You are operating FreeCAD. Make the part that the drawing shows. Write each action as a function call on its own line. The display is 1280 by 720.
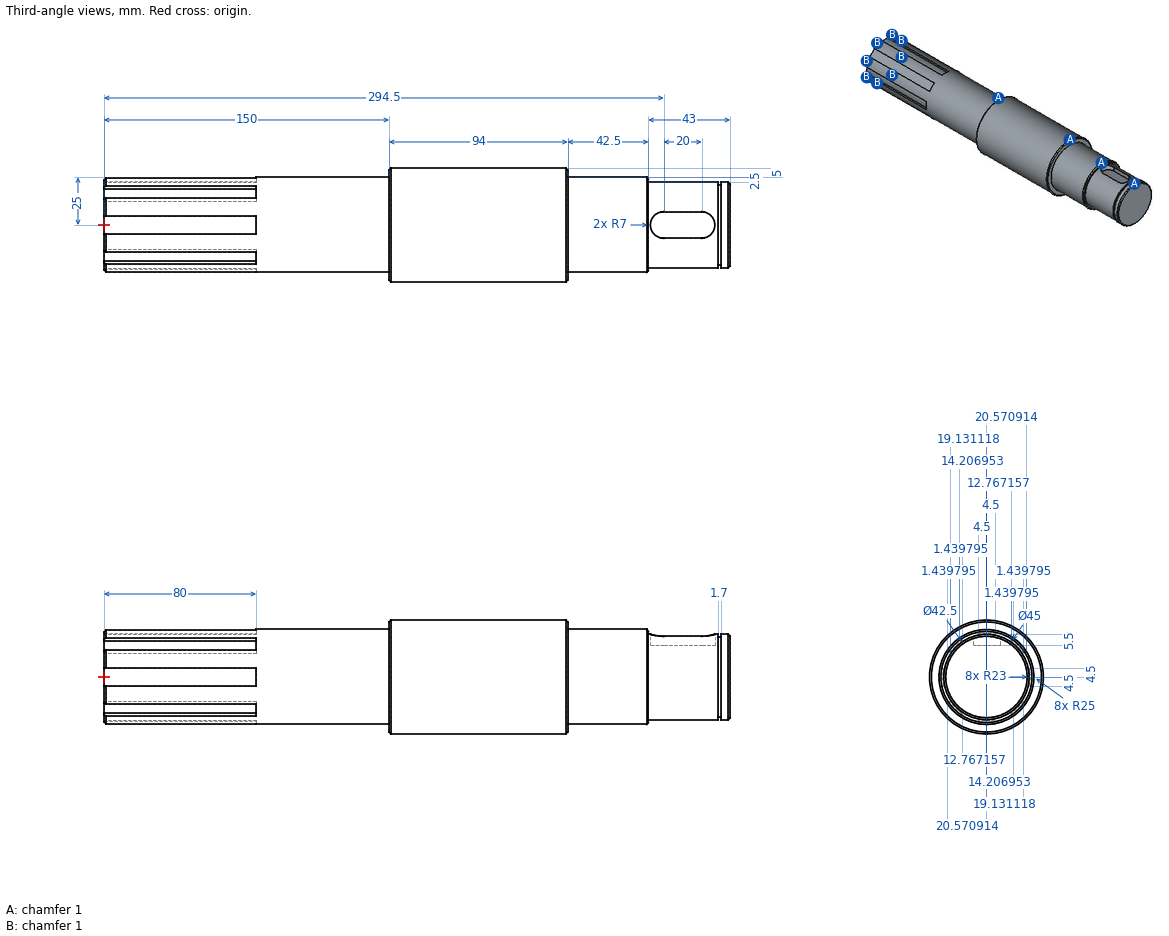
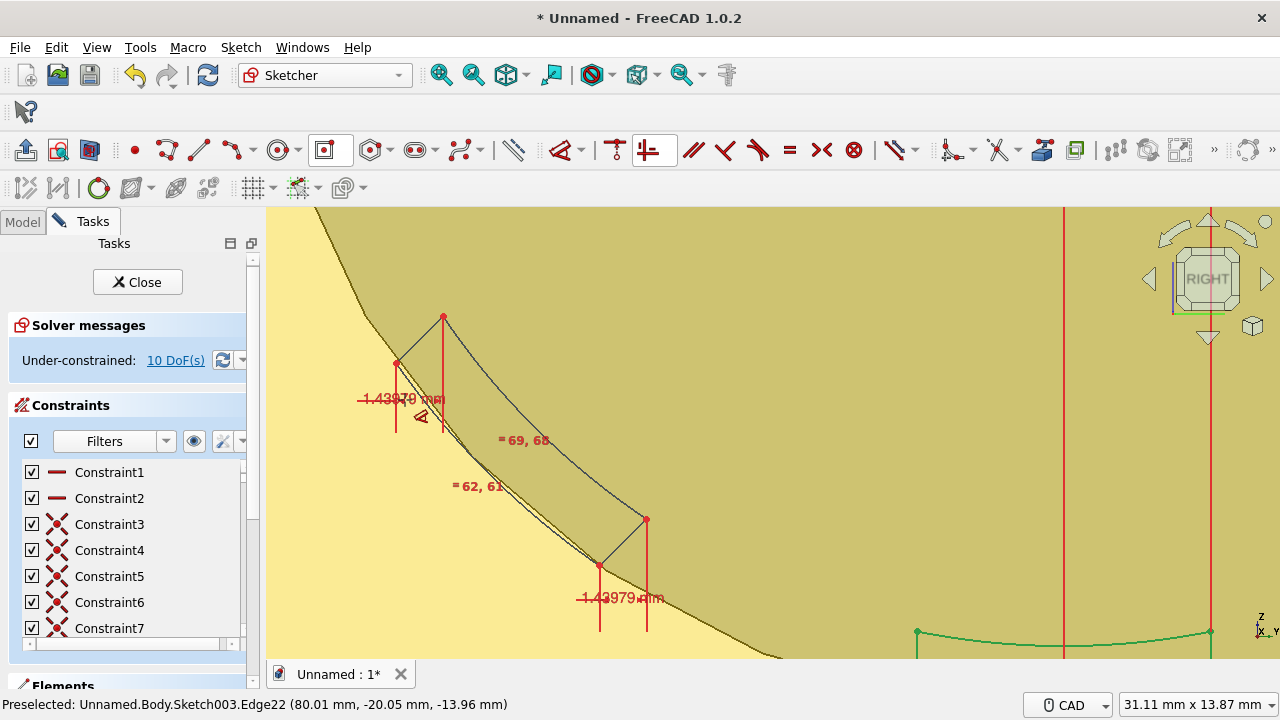
scroll(633, 539, down, 9)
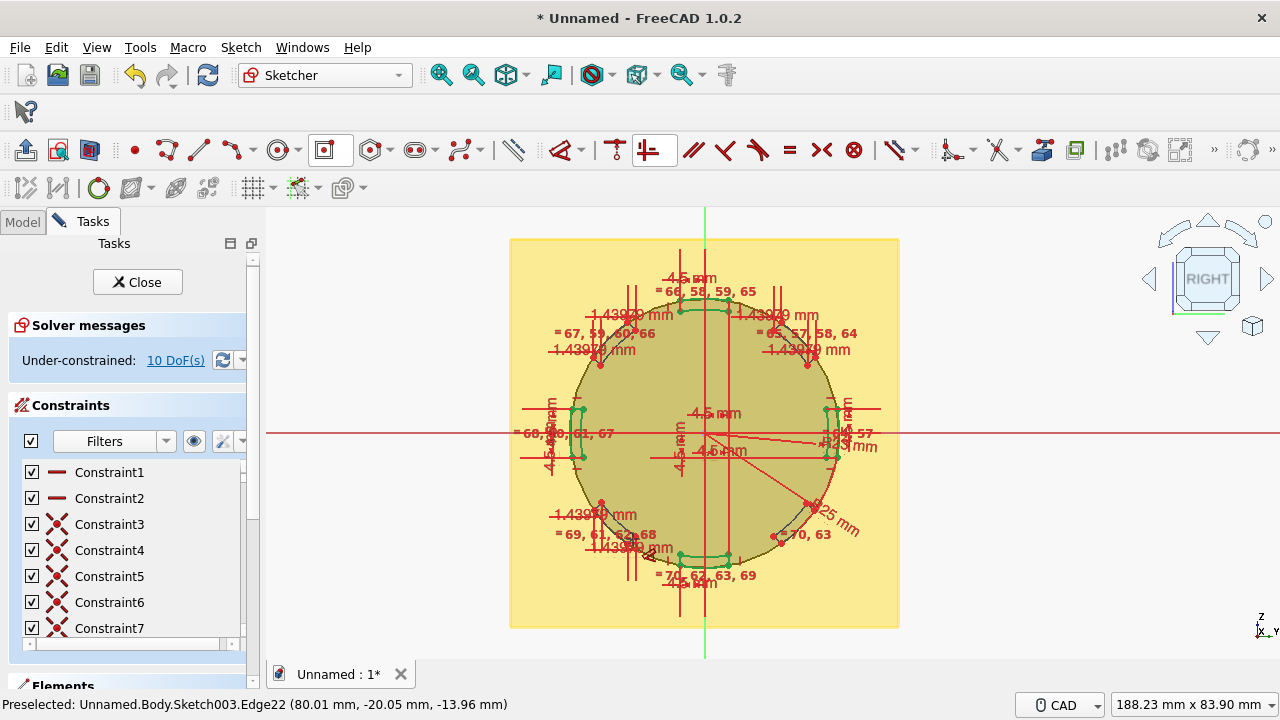
scroll(809, 506, up, 9)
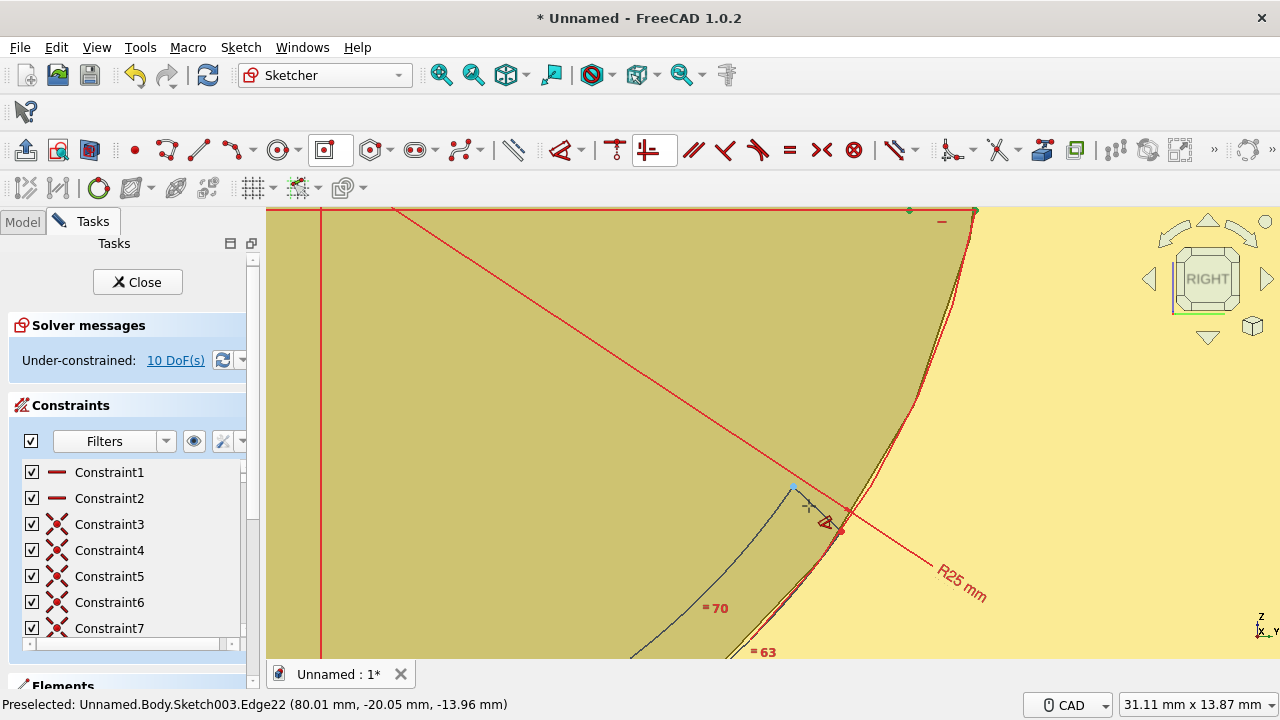
click(808, 500)
click(834, 566)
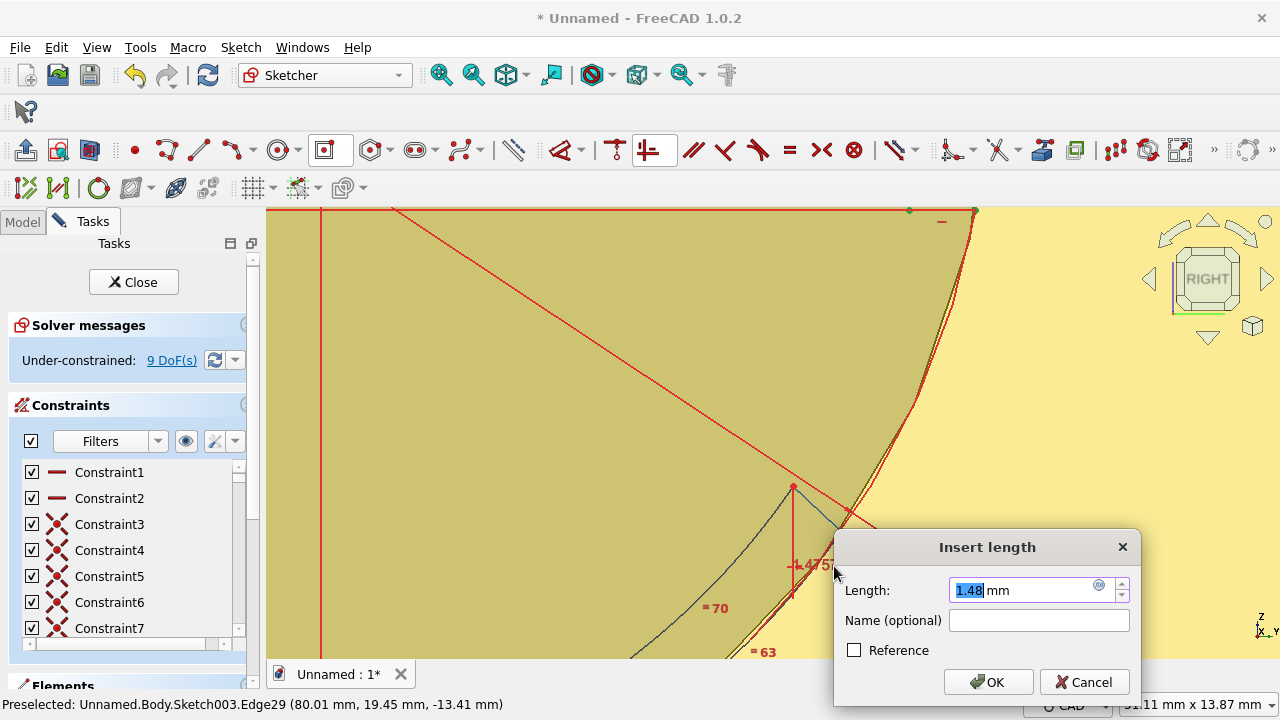
text(1.439795)
key(Return)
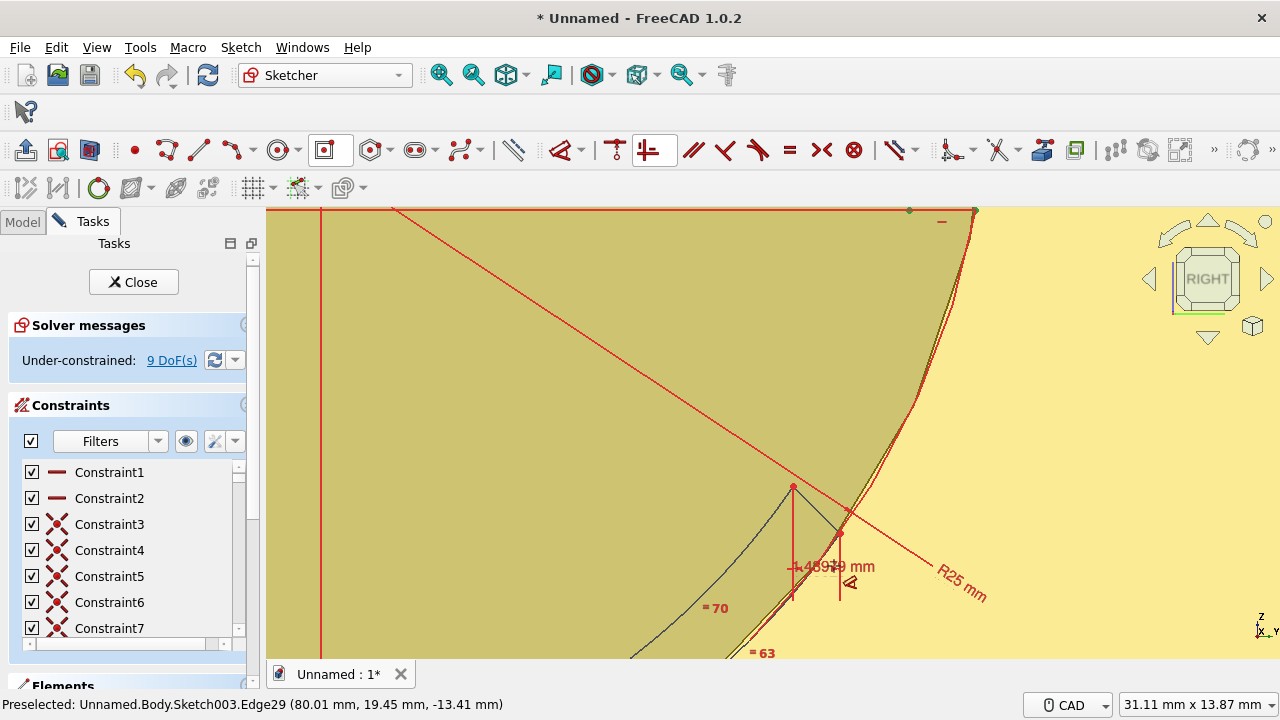
scroll(809, 506, down, 9)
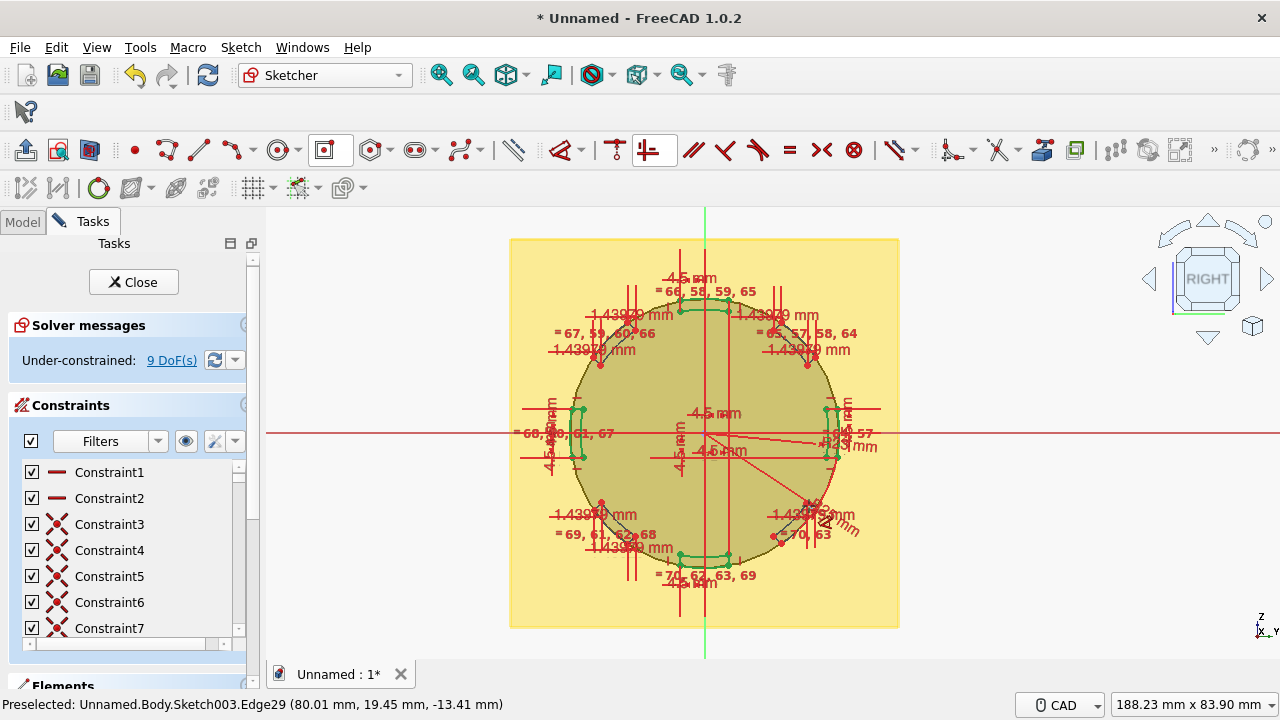
scroll(779, 542, up, 9)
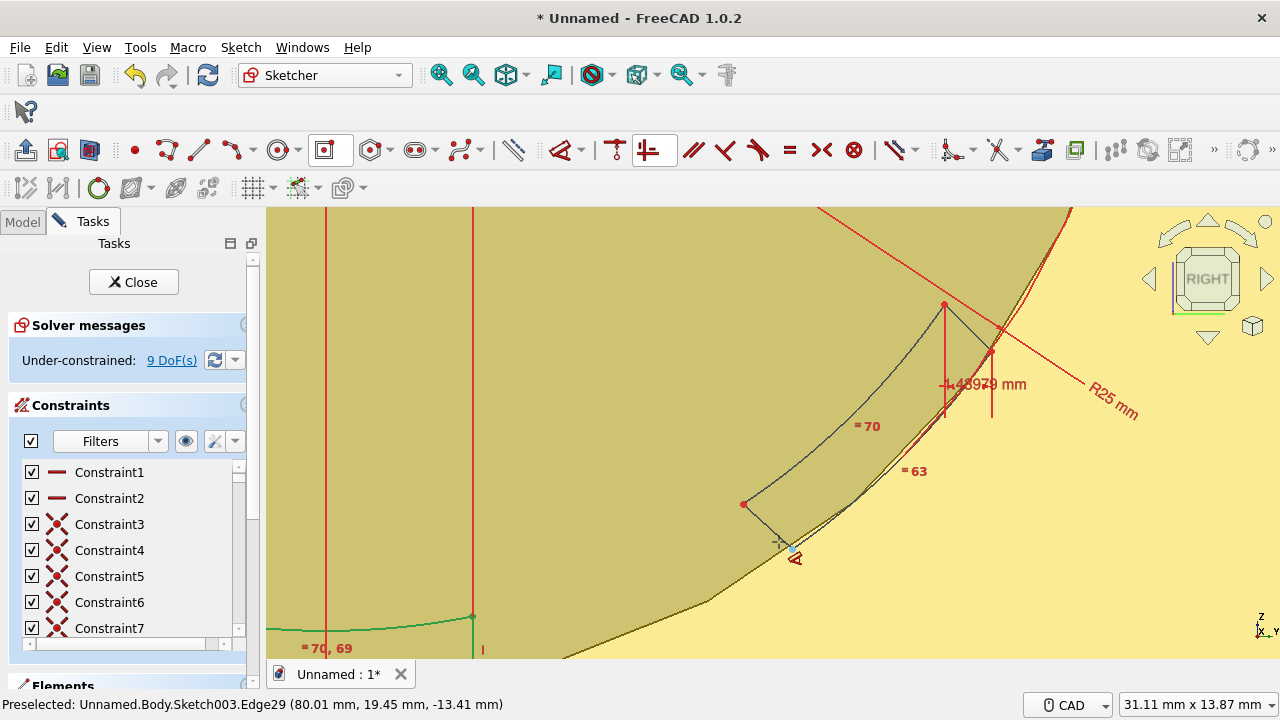
click(778, 536)
click(768, 583)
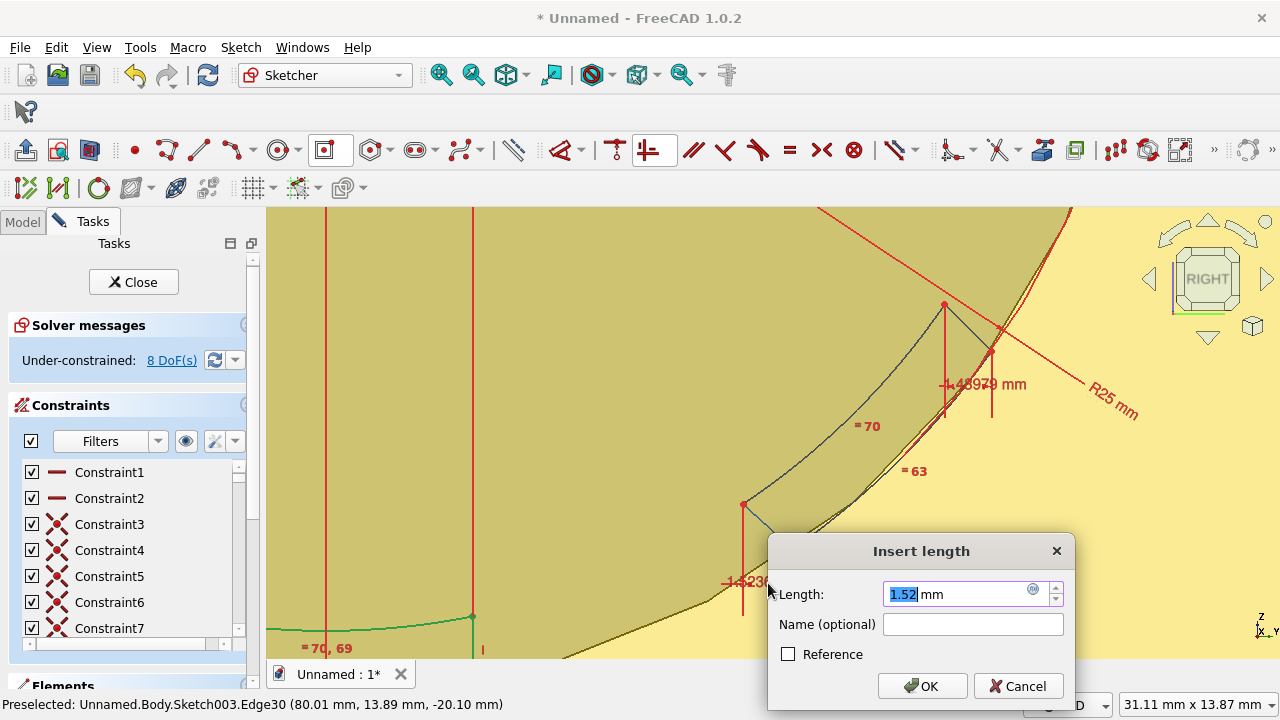
text(1.439795)
key(Return)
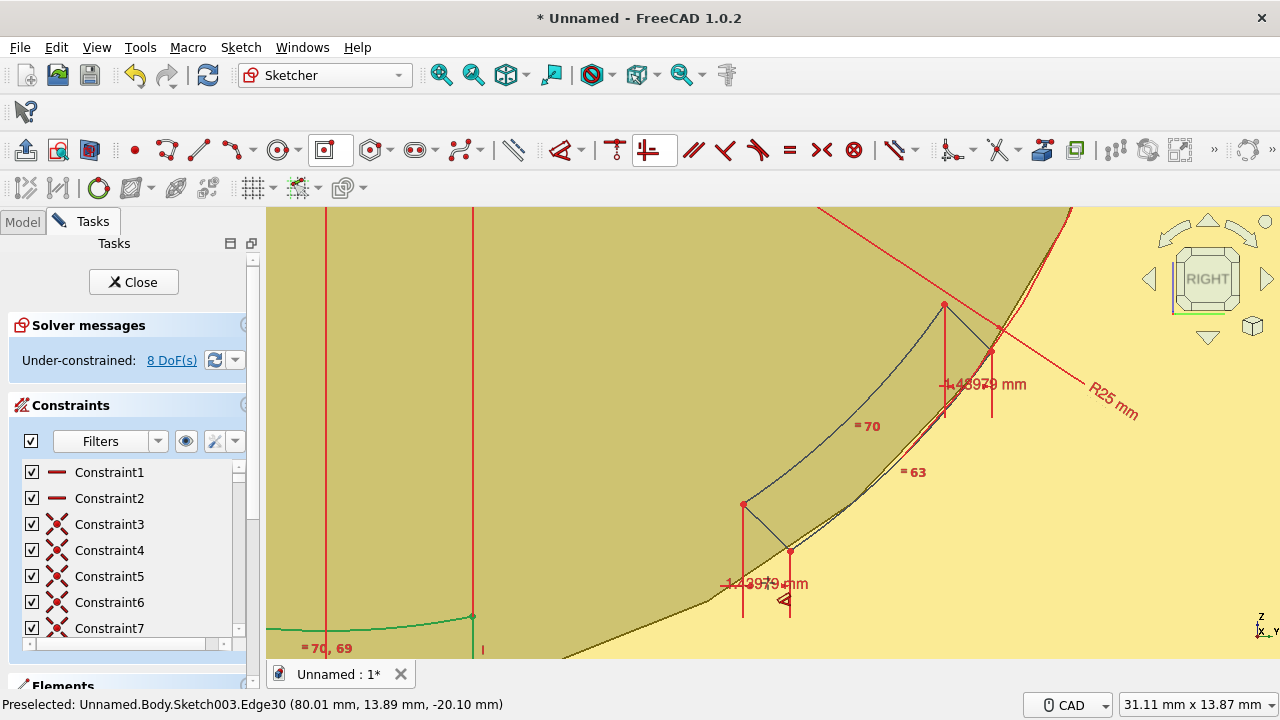
scroll(779, 542, down, 9)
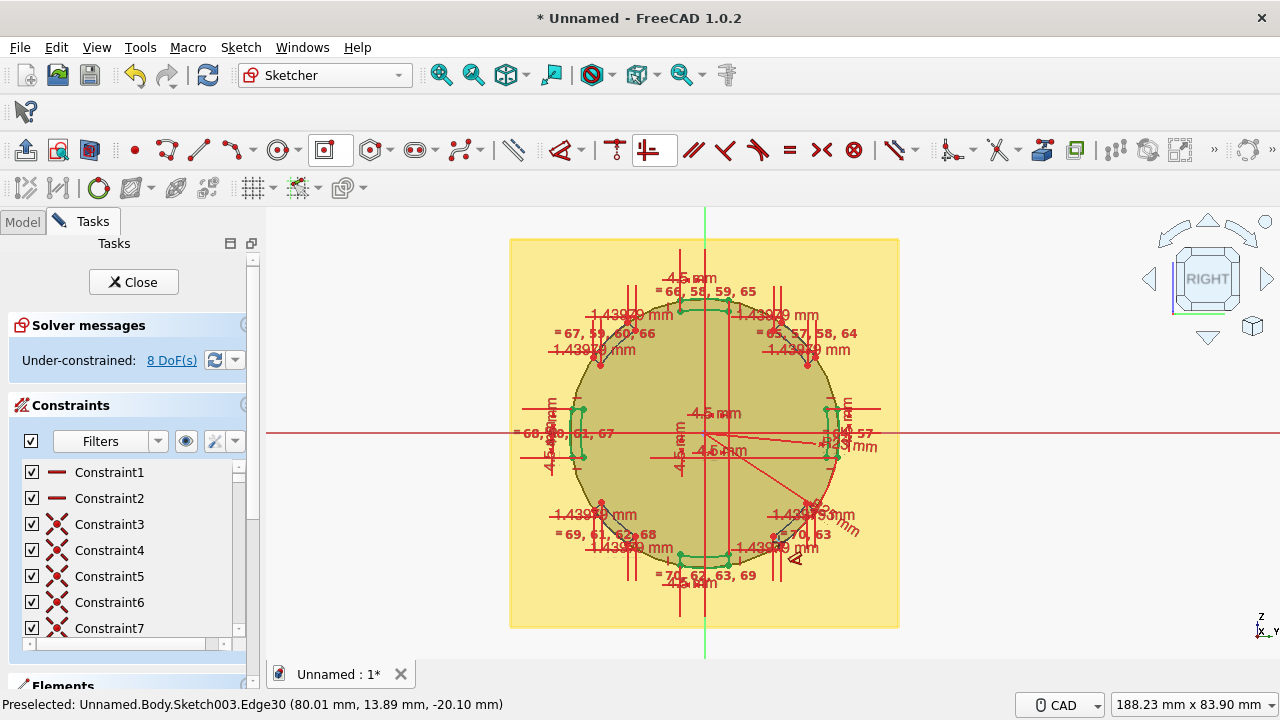
click(774, 331)
click(763, 297)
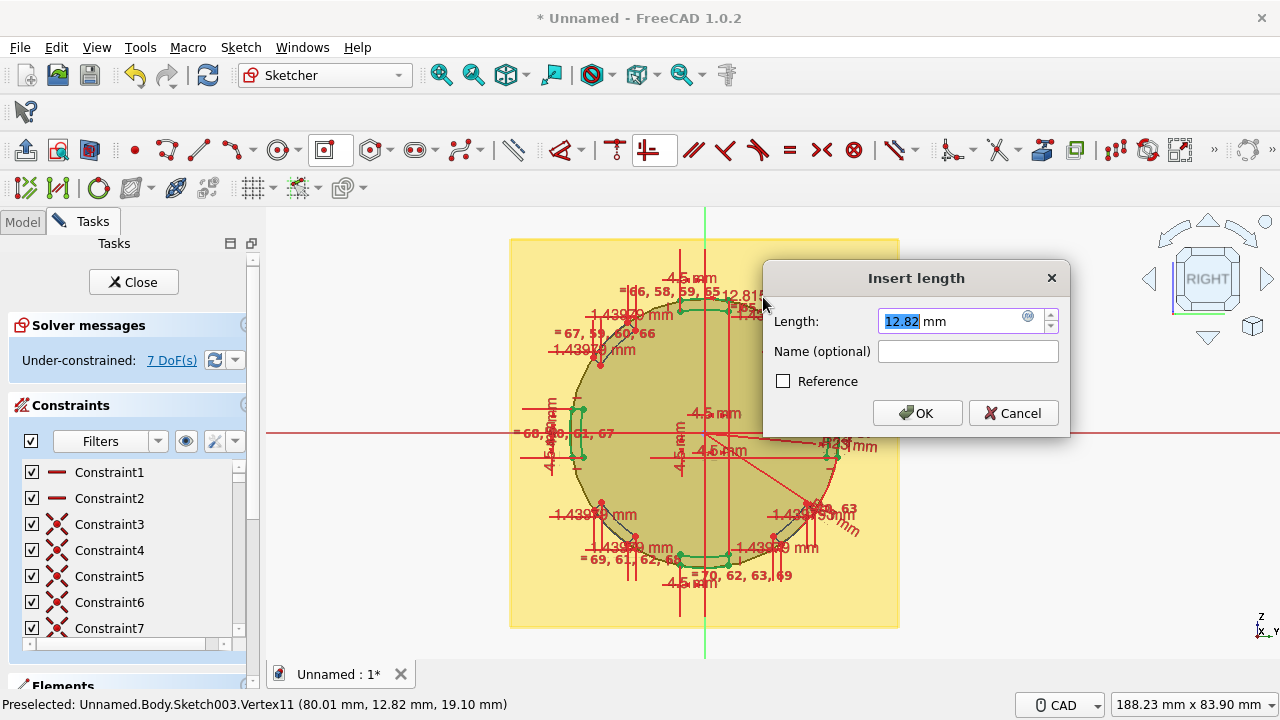
text(12.767157)
key(Return)